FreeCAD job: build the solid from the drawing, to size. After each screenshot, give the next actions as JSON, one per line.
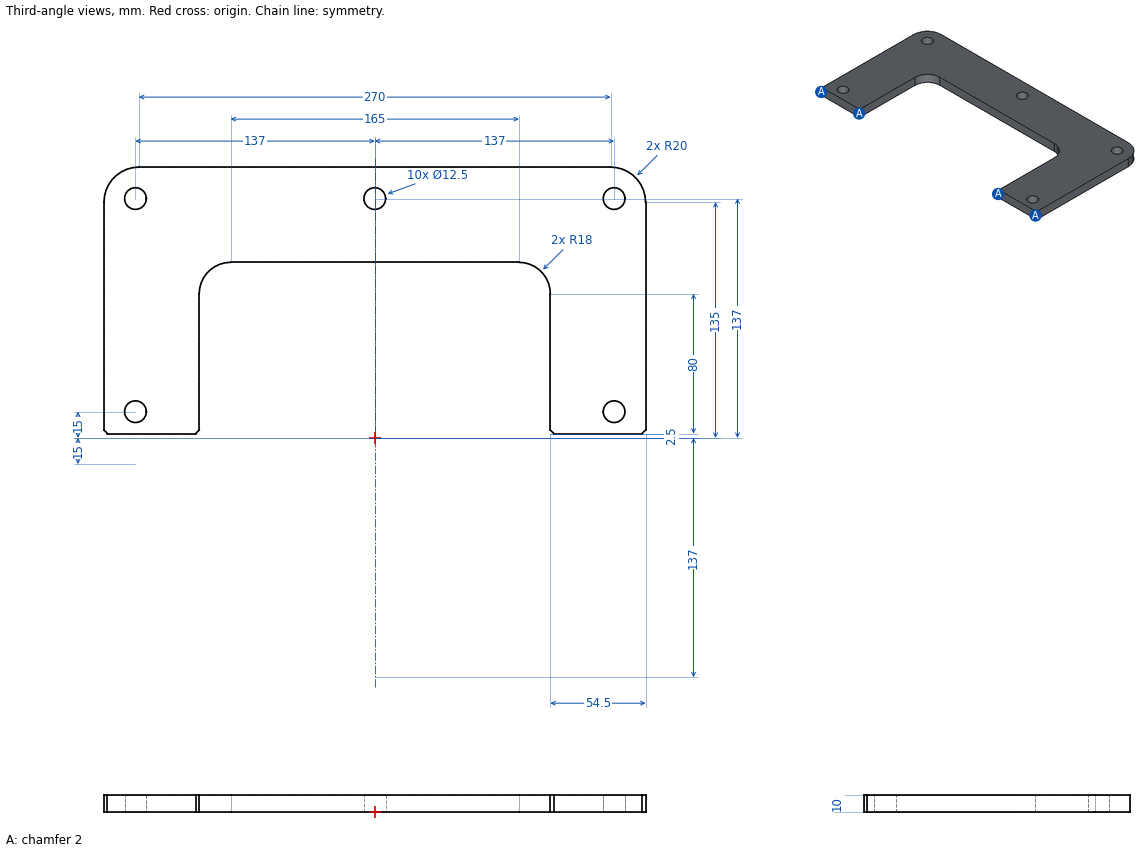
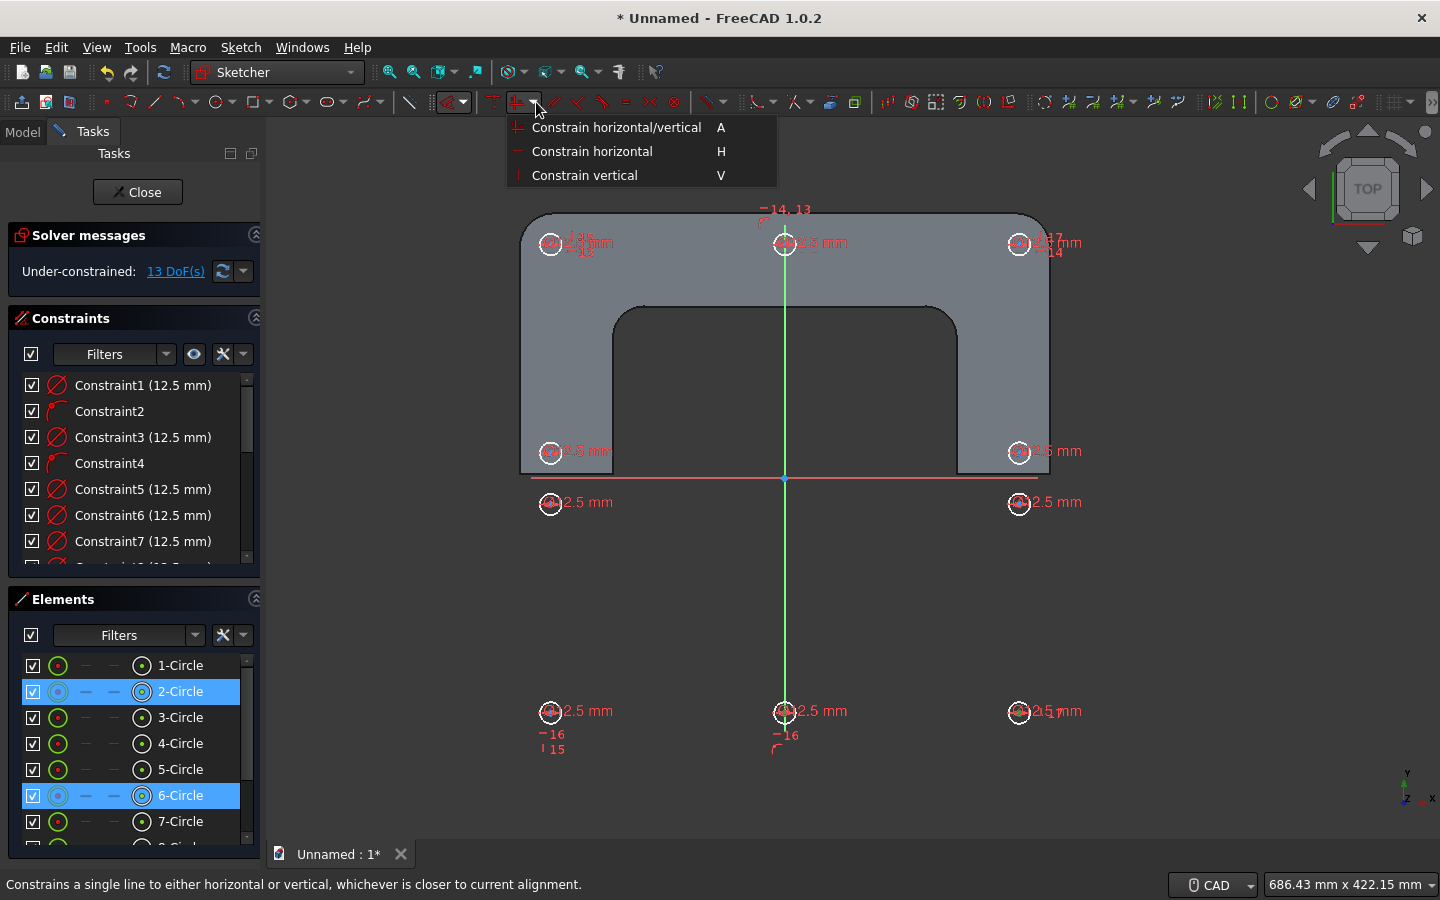
{"action": "left_click", "coordinate": [642, 151]}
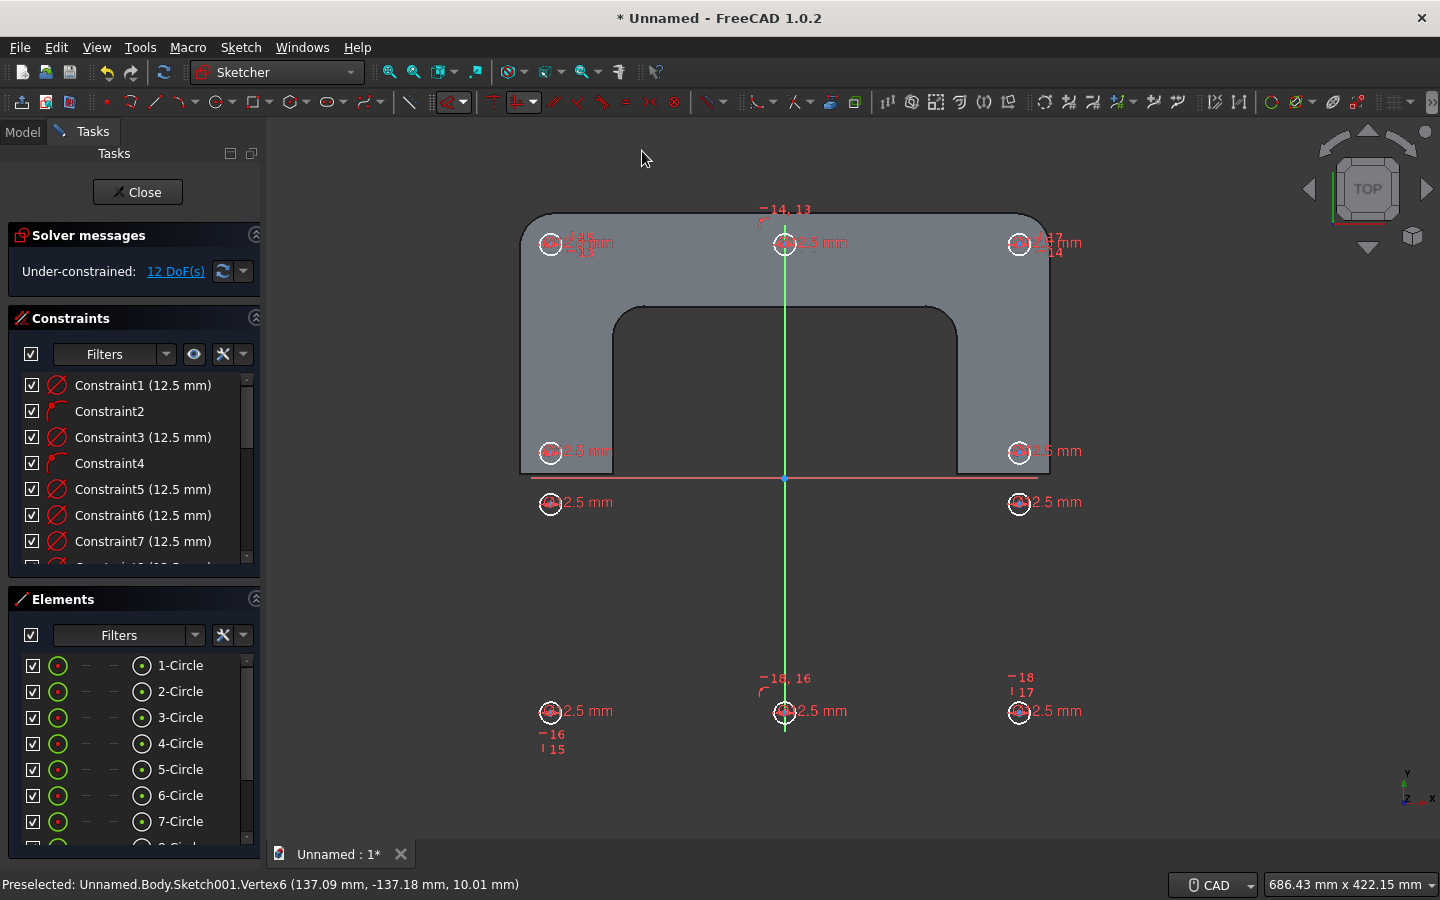
{"action": "left_click", "coordinate": [551, 245]}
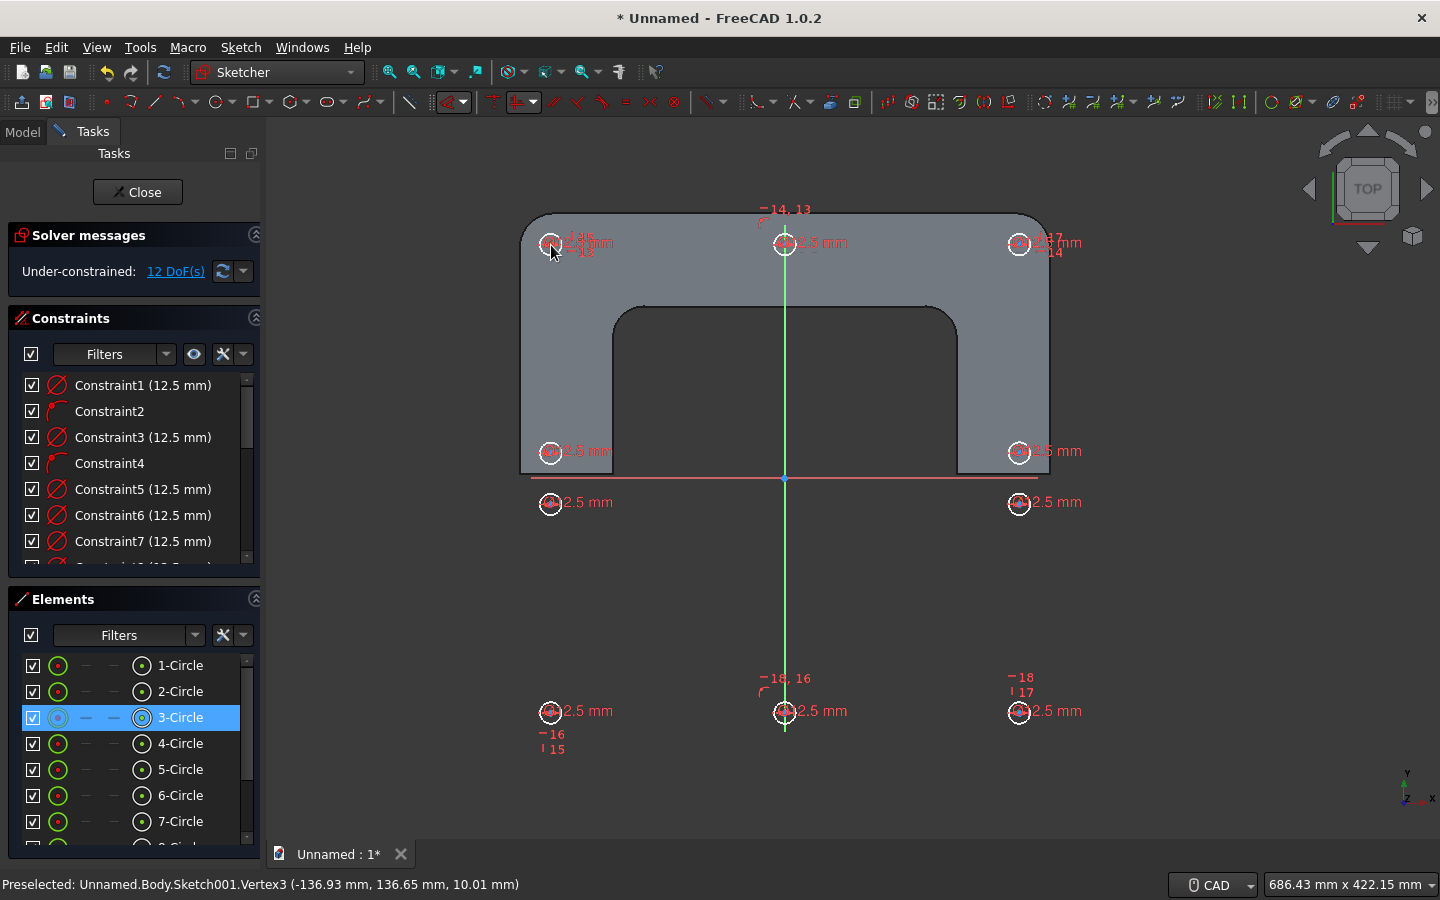
{"action": "left_click", "coordinate": [551, 453]}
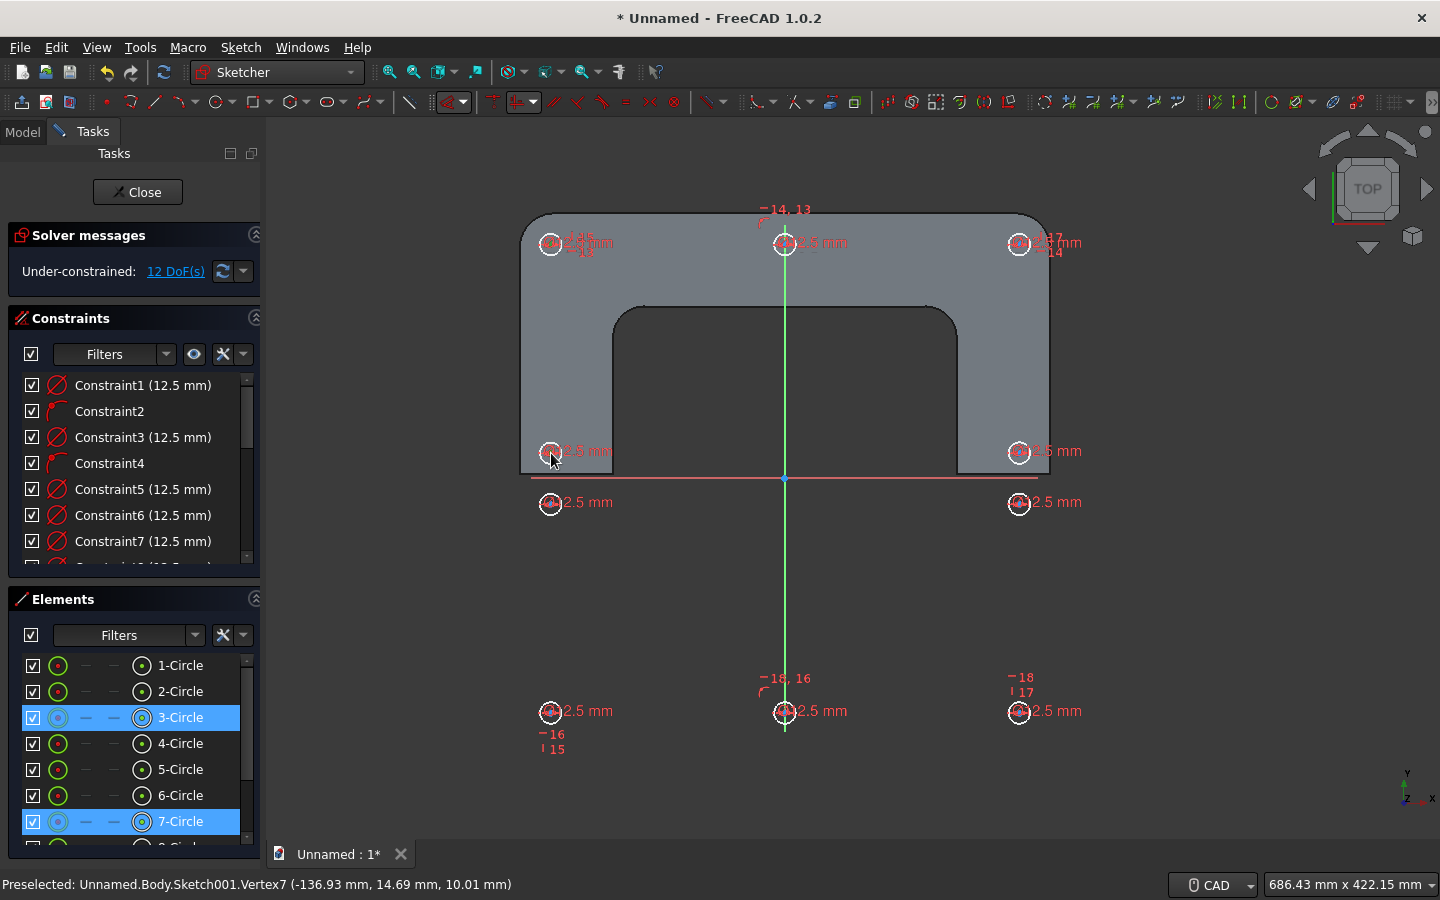
{"action": "key", "text": "v"}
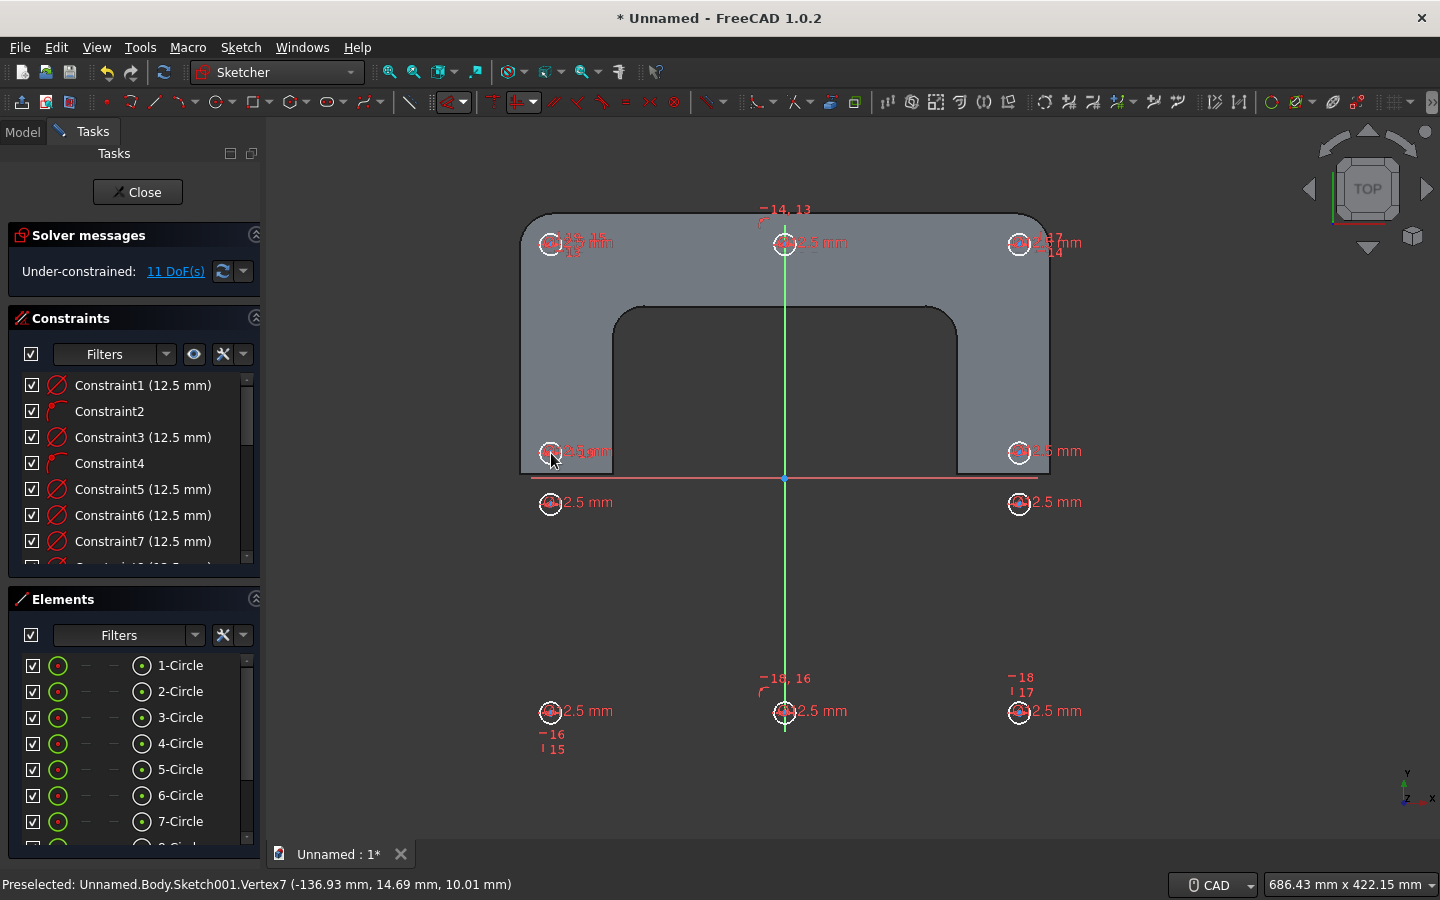
{"action": "left_click", "coordinate": [551, 453]}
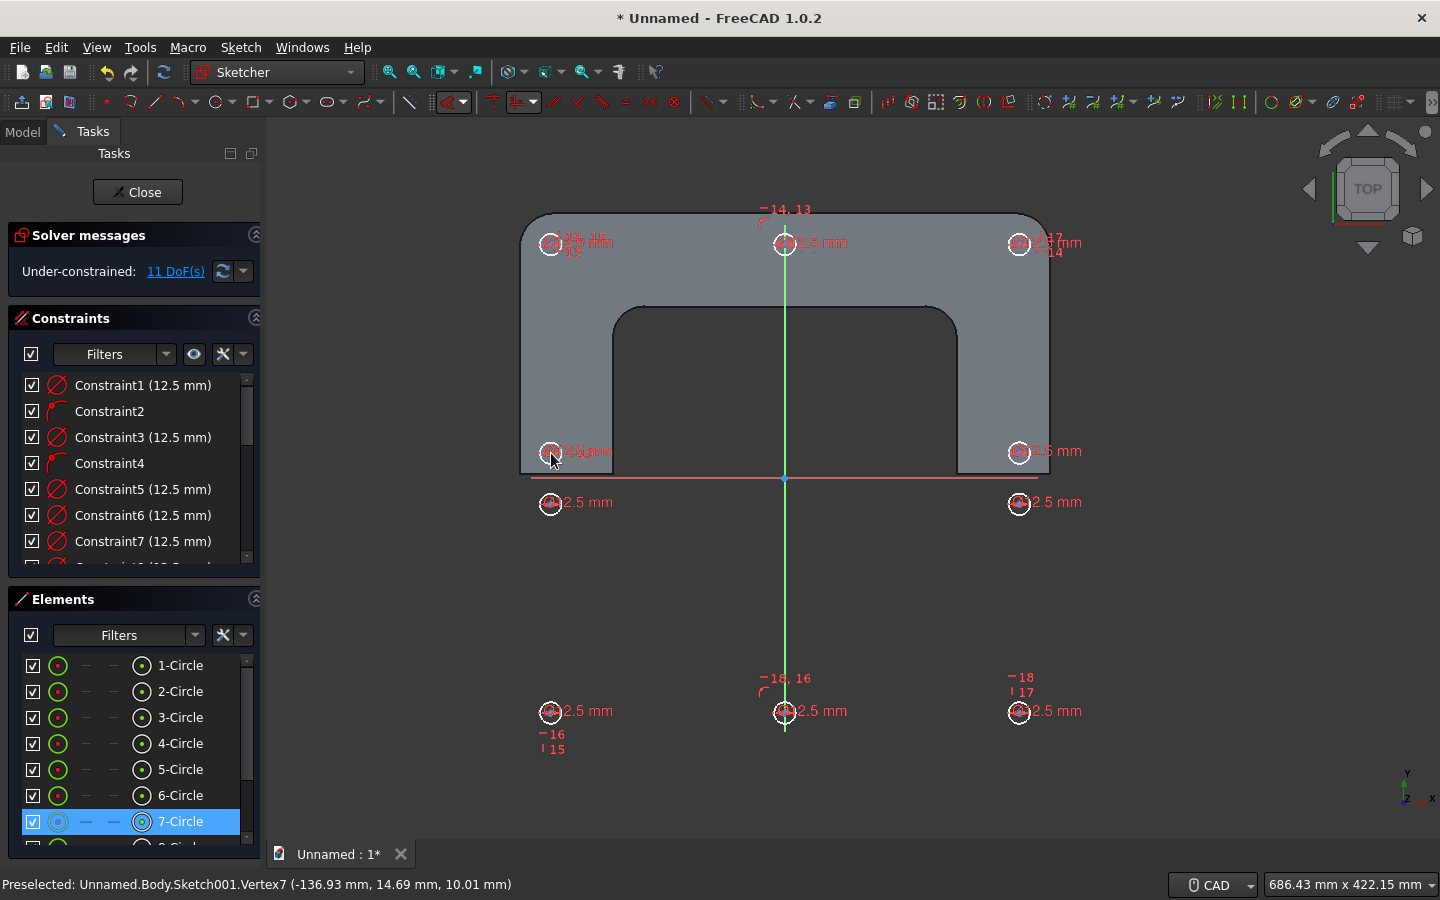
{"action": "left_click", "coordinate": [551, 504]}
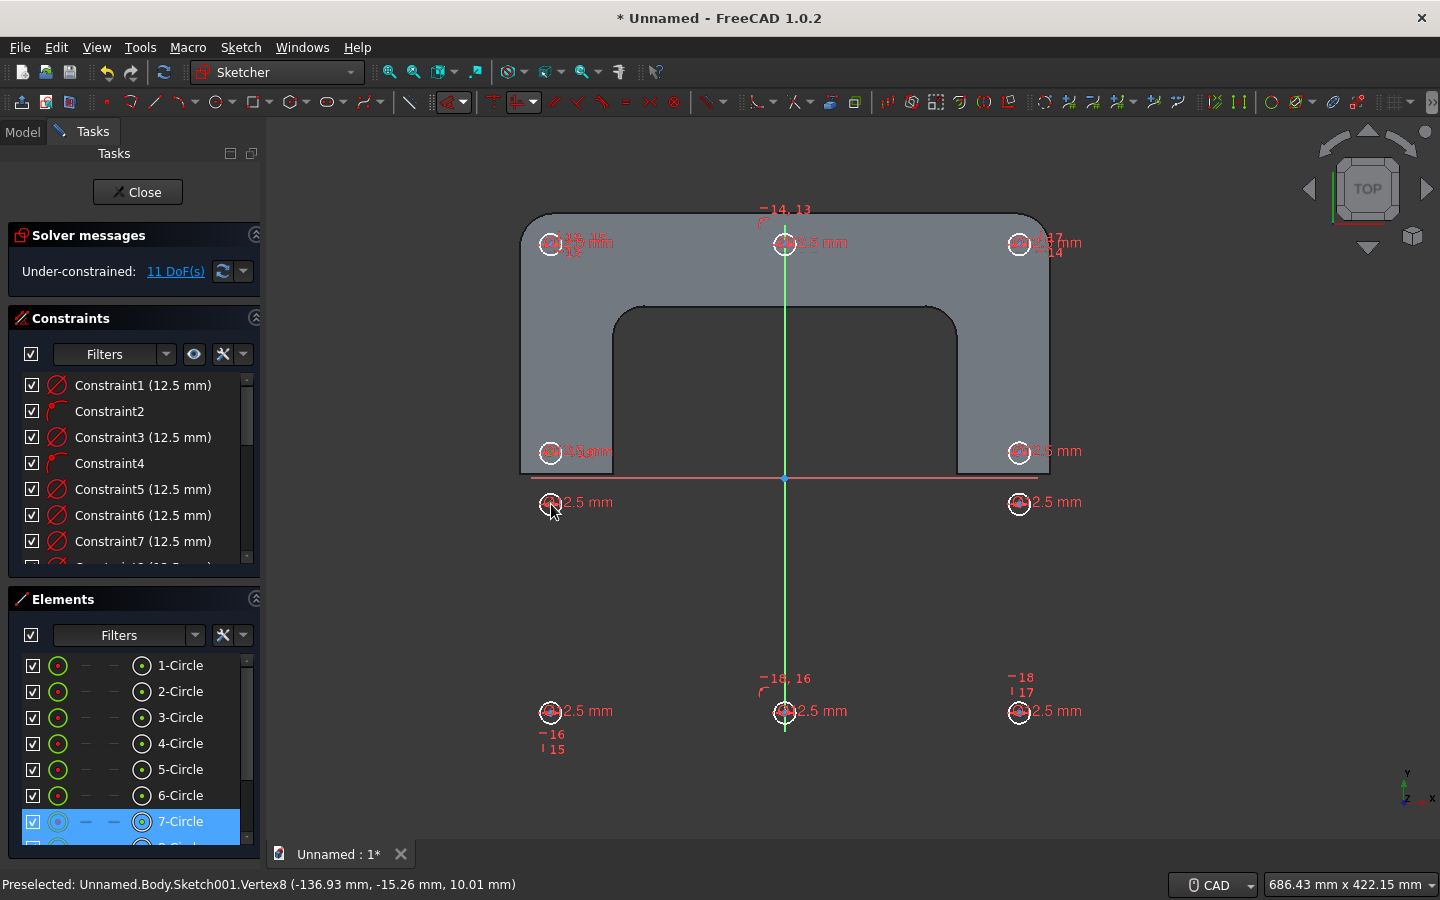
{"action": "key", "text": "v"}